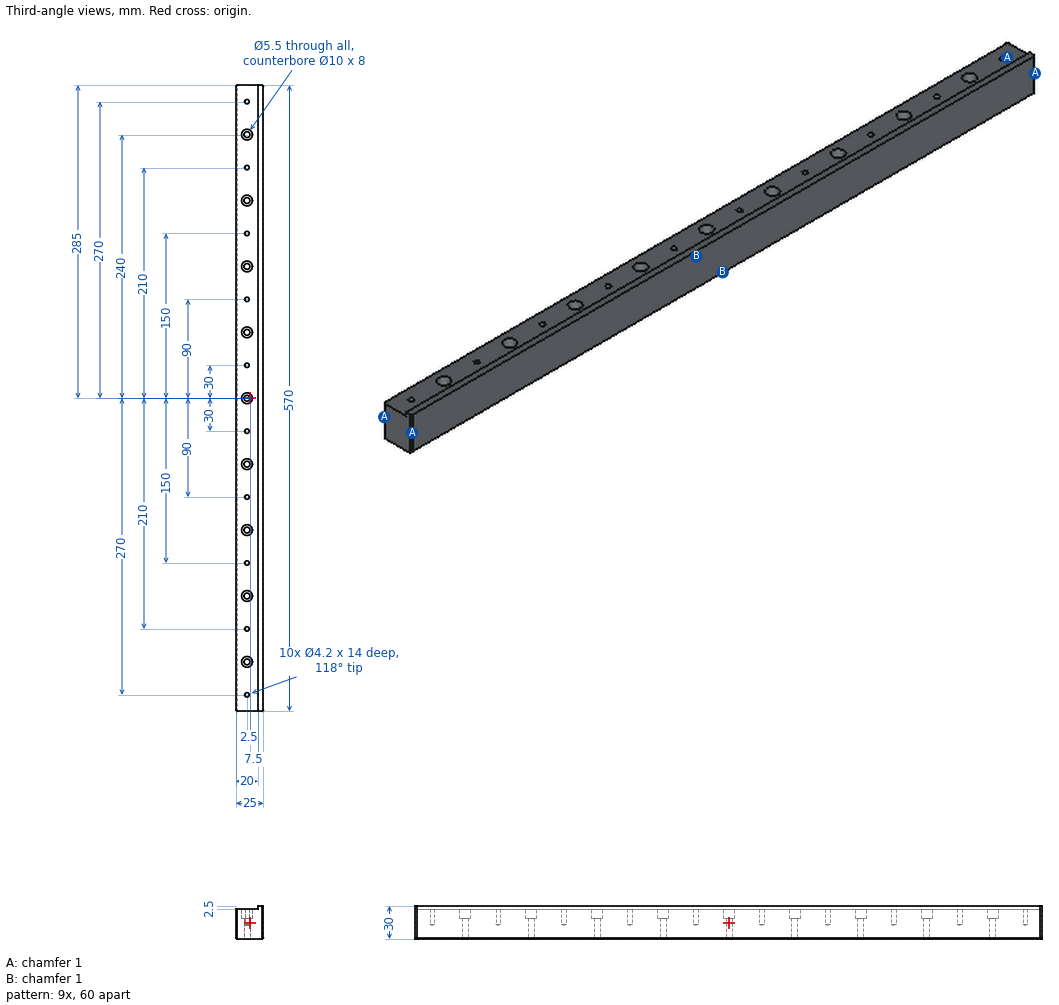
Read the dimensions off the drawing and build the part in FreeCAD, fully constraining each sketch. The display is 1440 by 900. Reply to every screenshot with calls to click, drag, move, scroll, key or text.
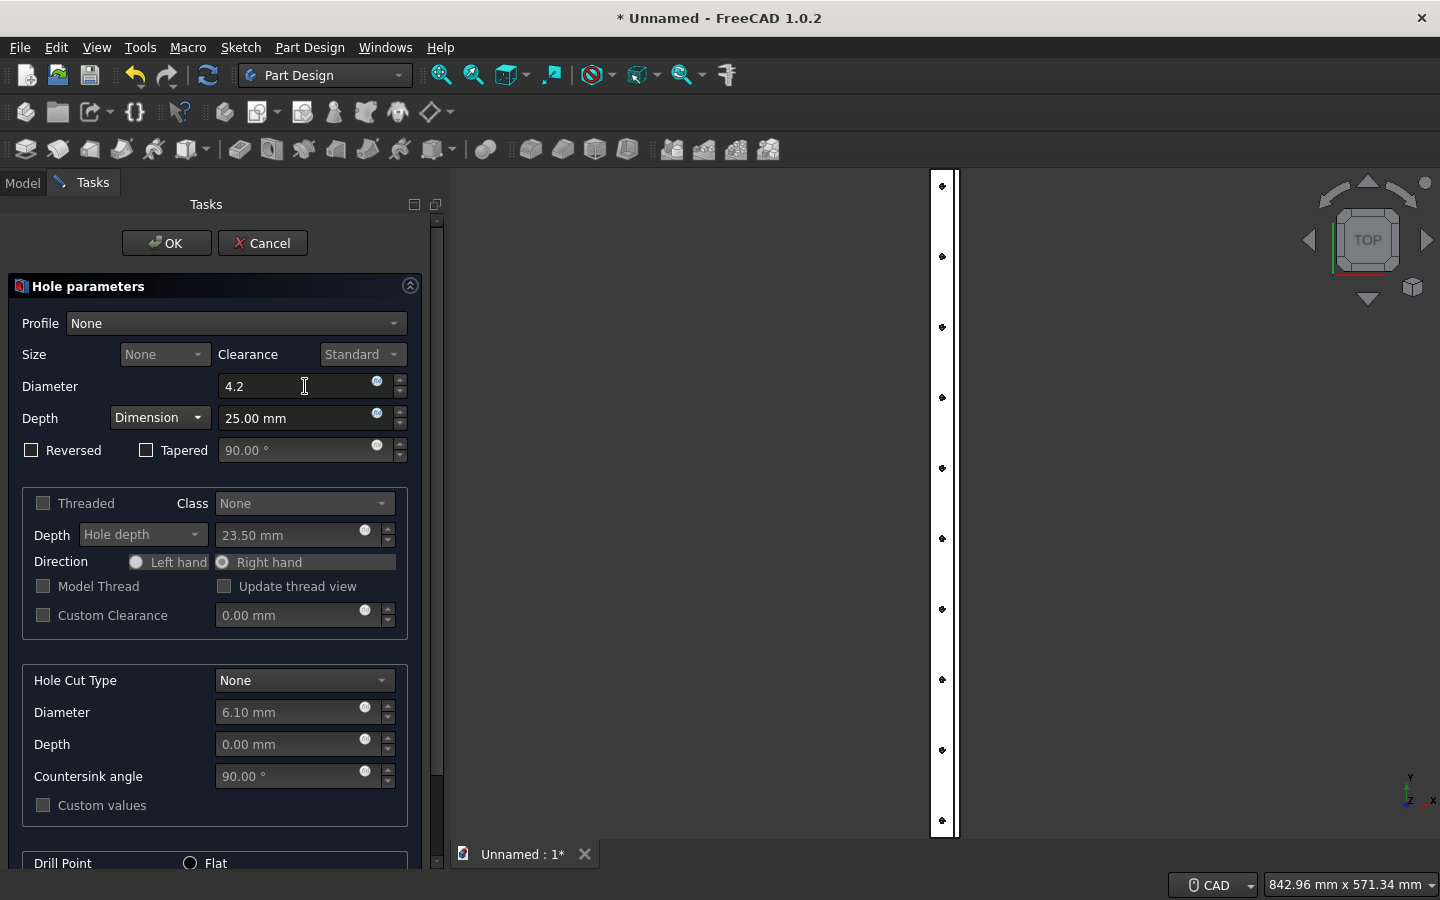
triple_click(305, 418)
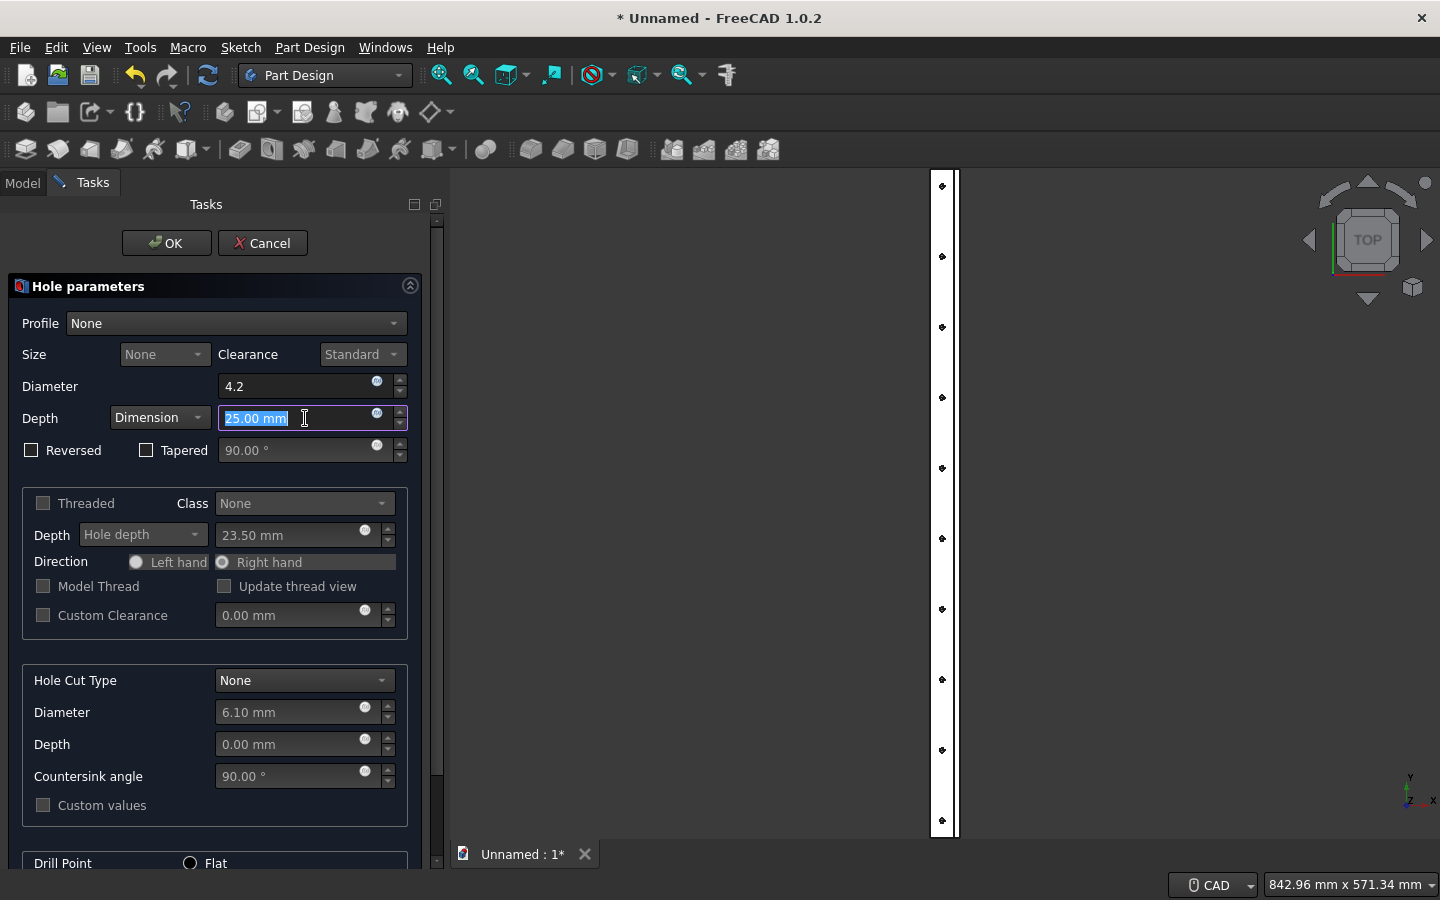
text(14)
key(Tab)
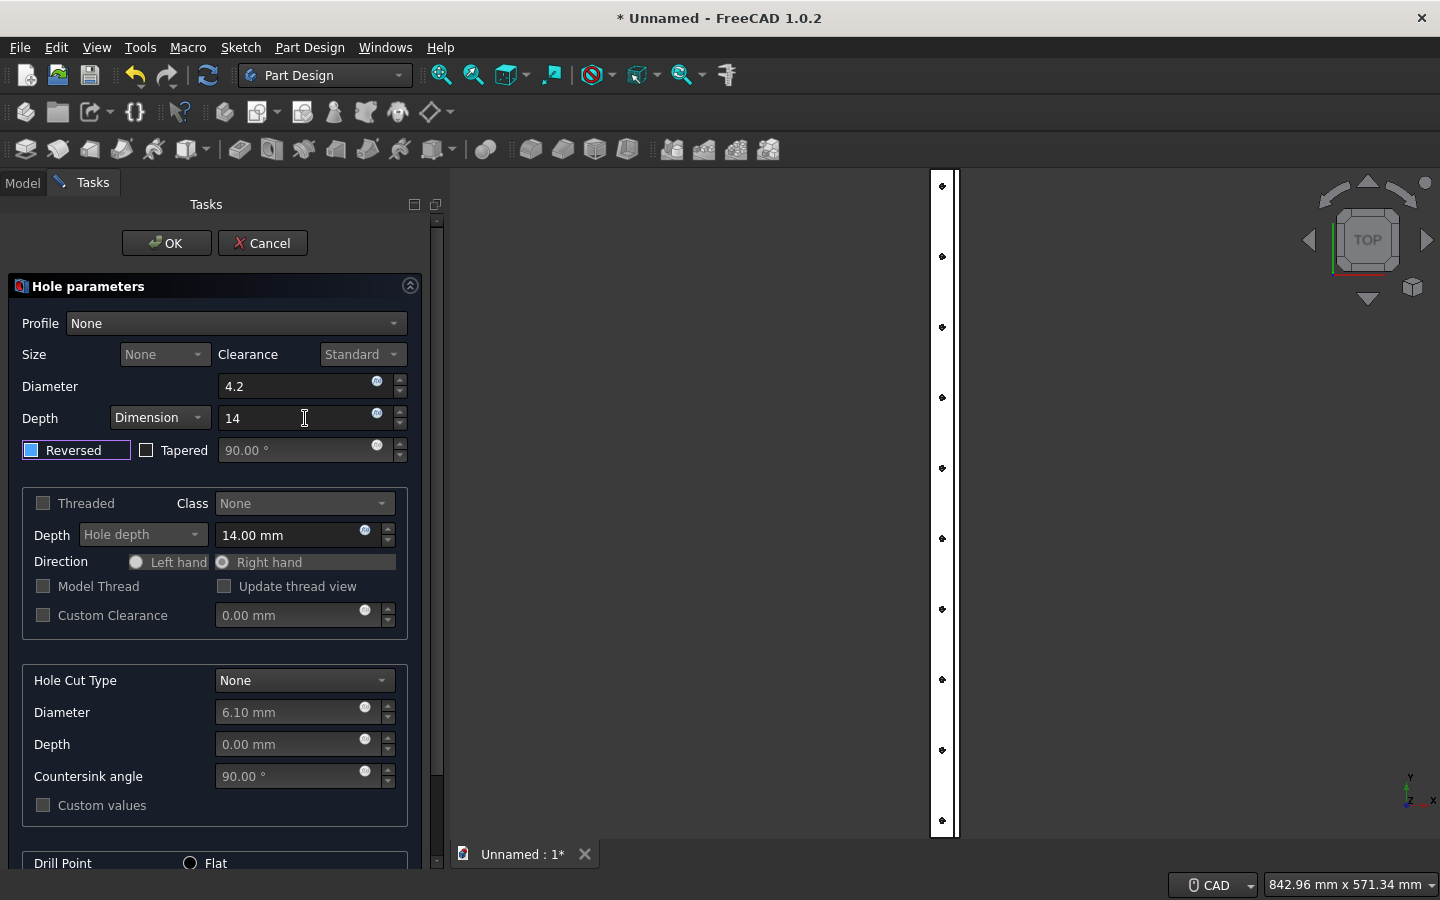
click(167, 243)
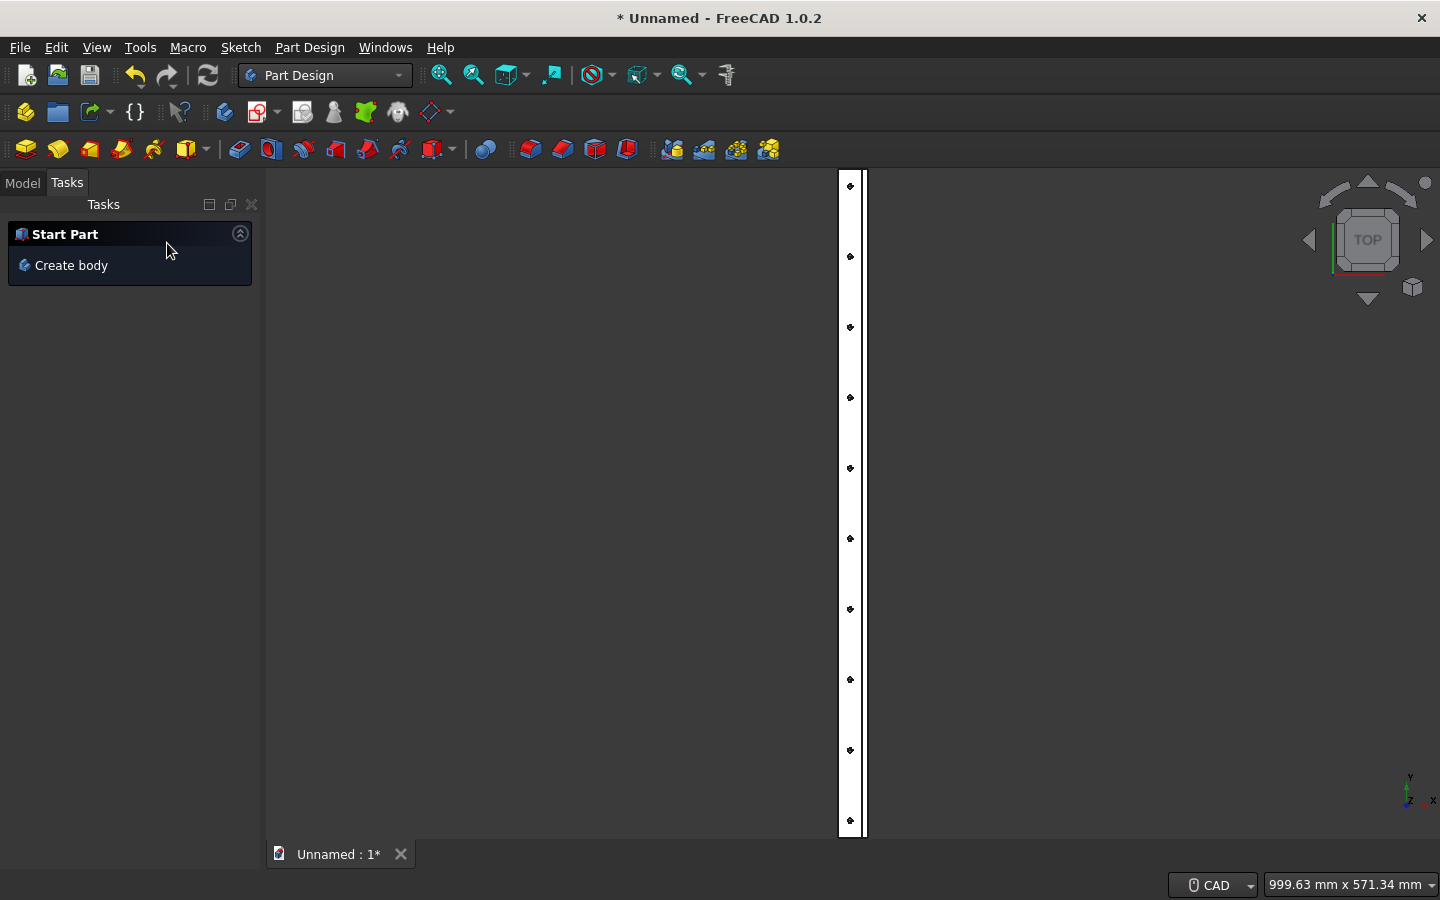
click(850, 216)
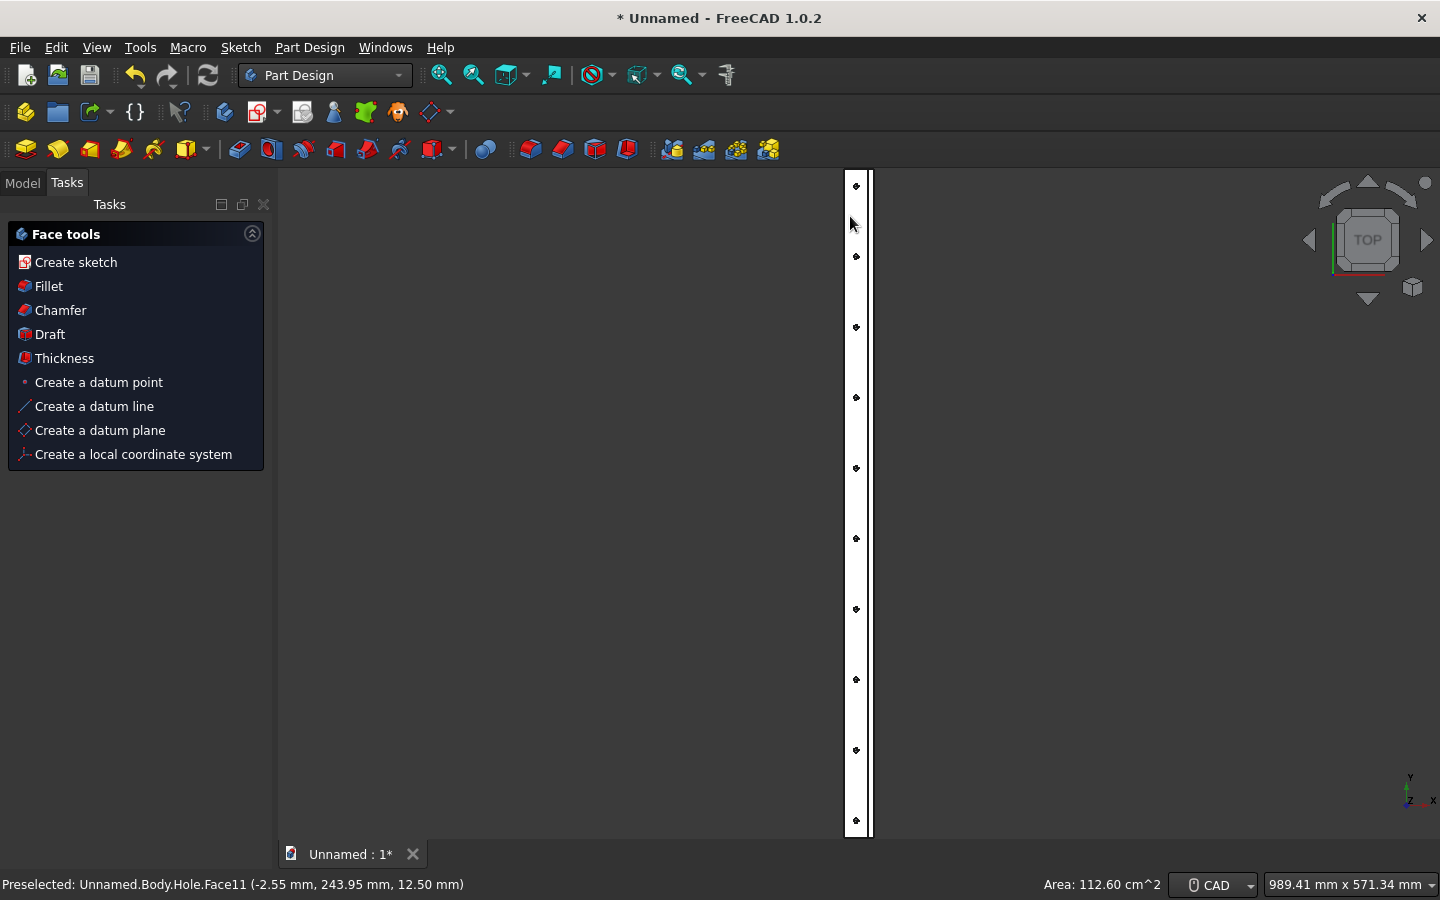
click(258, 112)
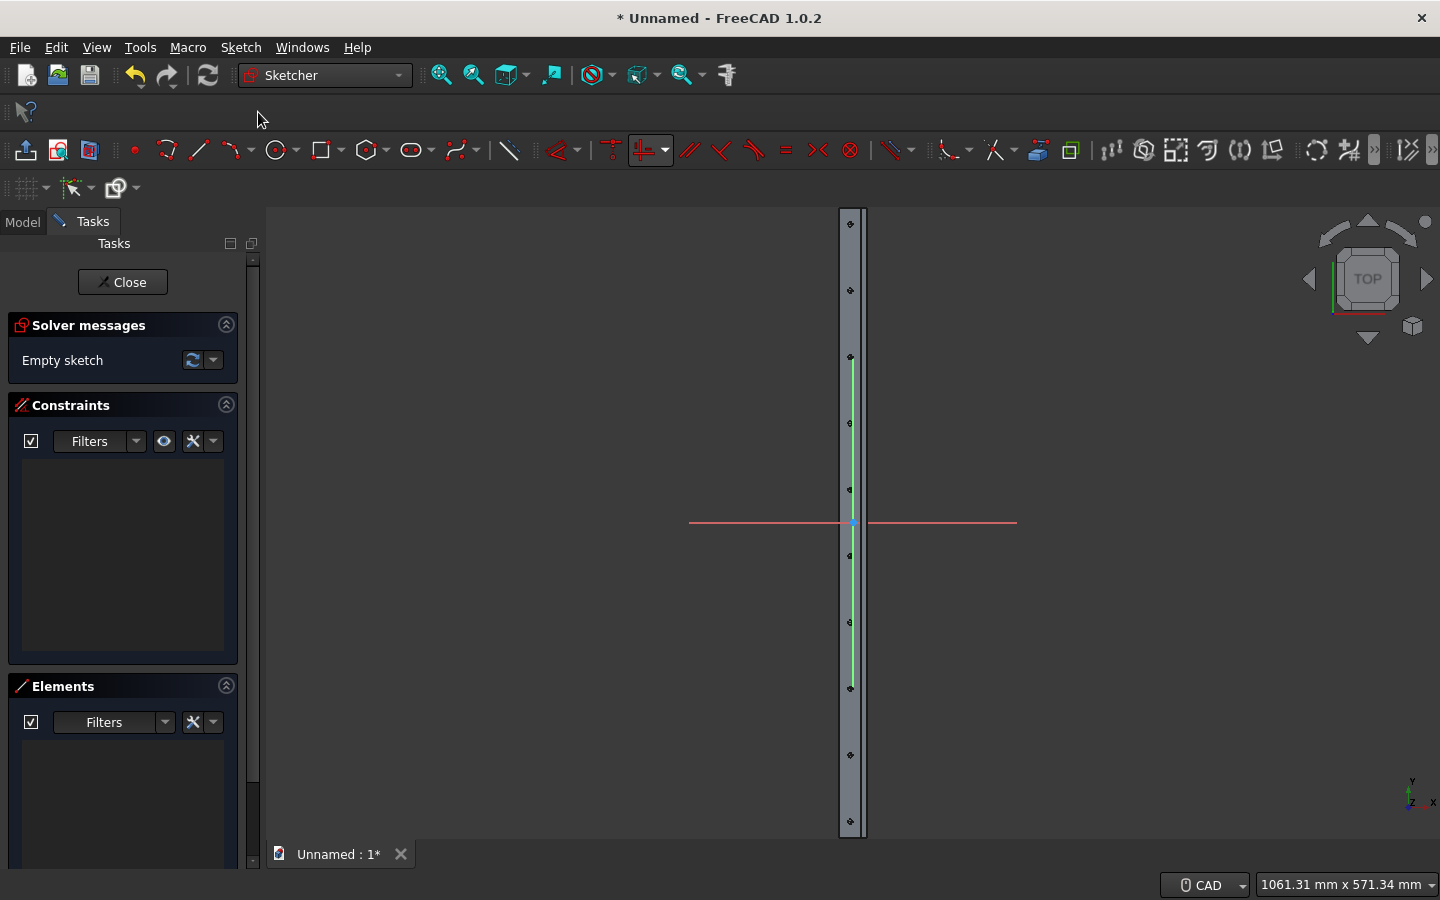
scroll(854, 244, up, 15)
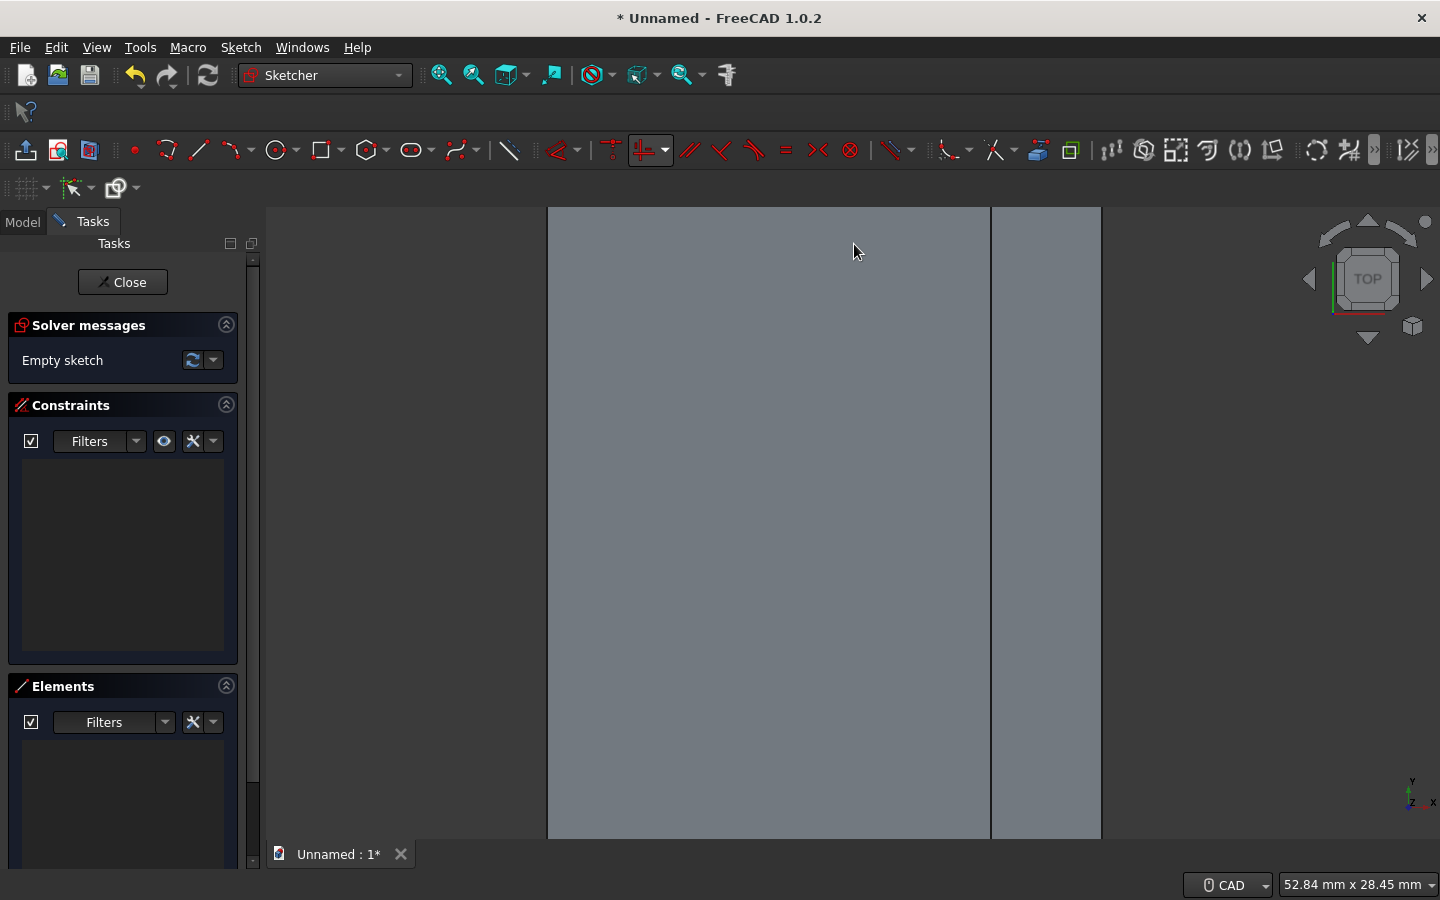
scroll(762, 511, up, 6)